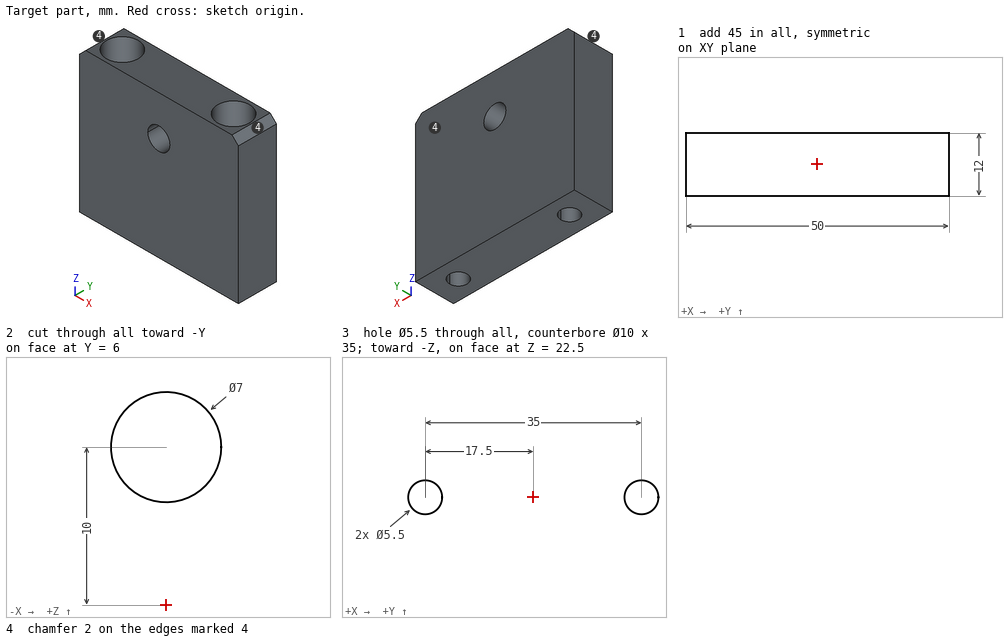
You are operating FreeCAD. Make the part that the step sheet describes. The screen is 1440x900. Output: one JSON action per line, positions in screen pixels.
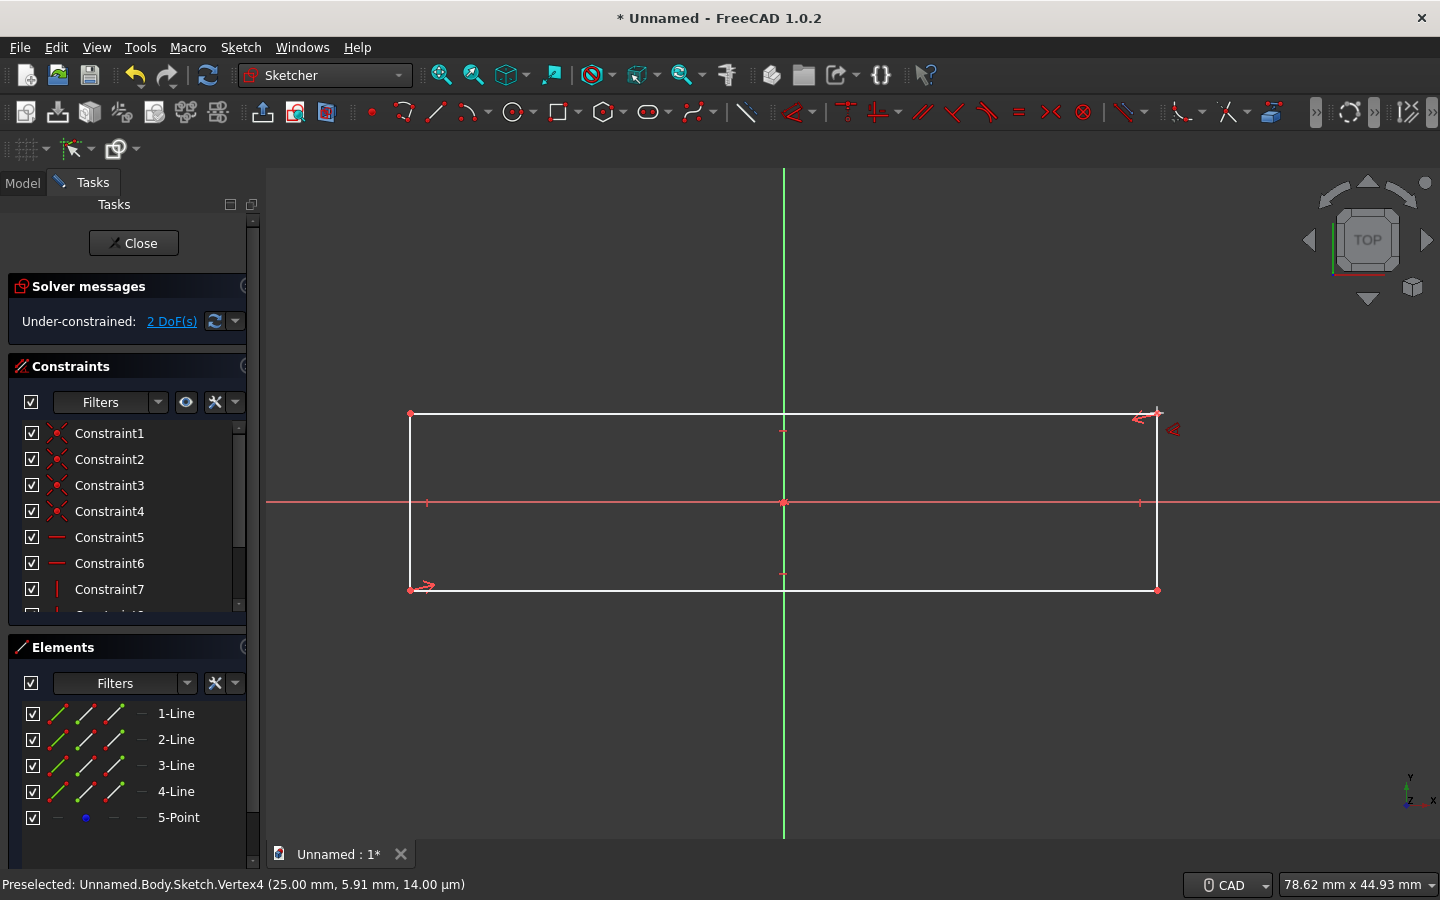
{"action": "left_click", "coordinate": [634, 591]}
{"action": "left_click", "coordinate": [612, 625]}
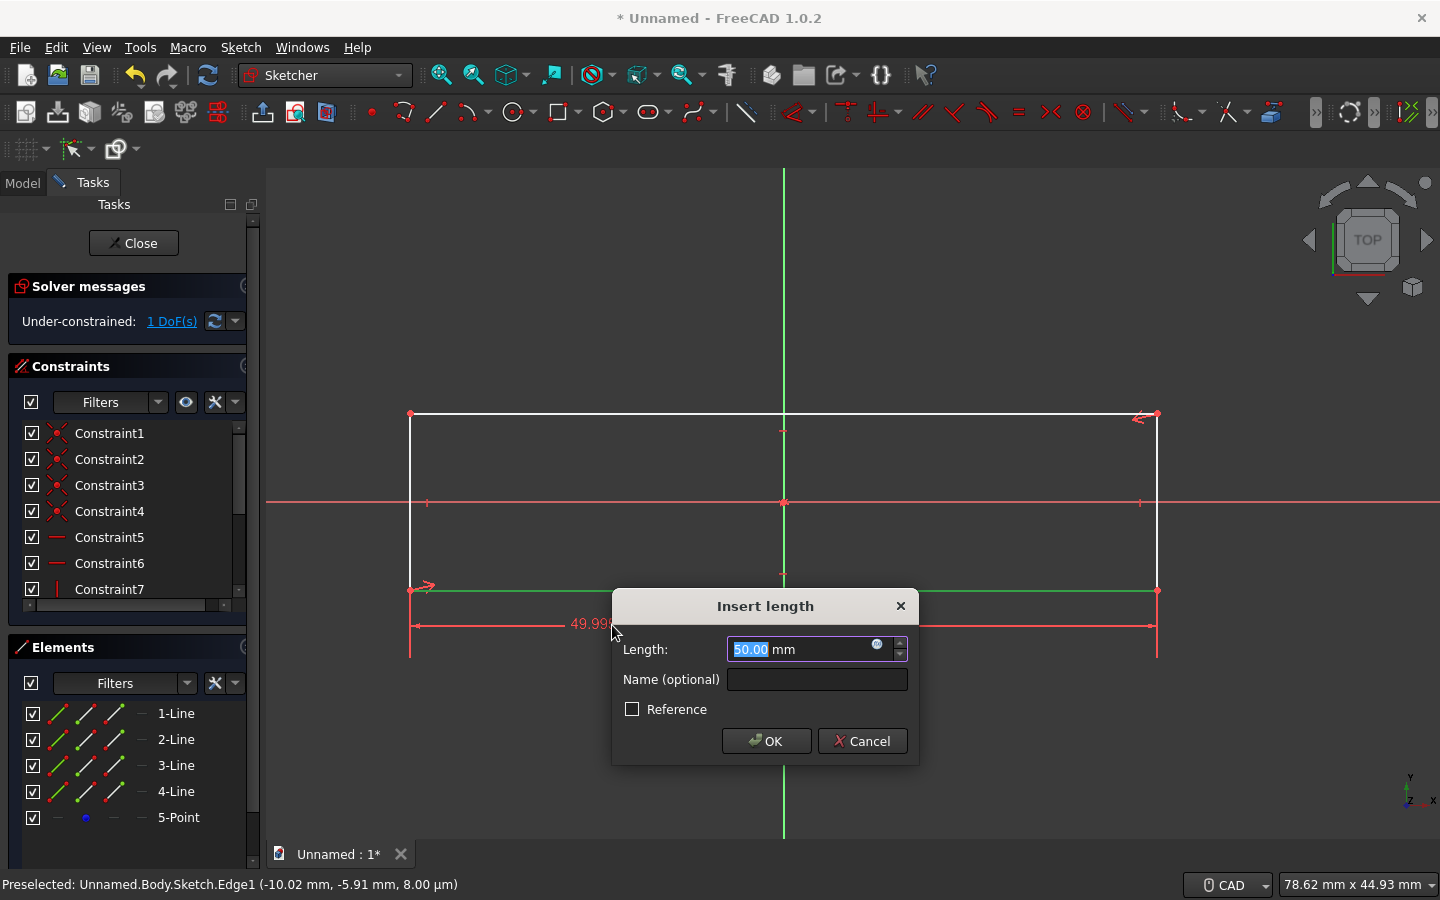
{"action": "type", "text": "50"}
{"action": "key", "text": "Return"}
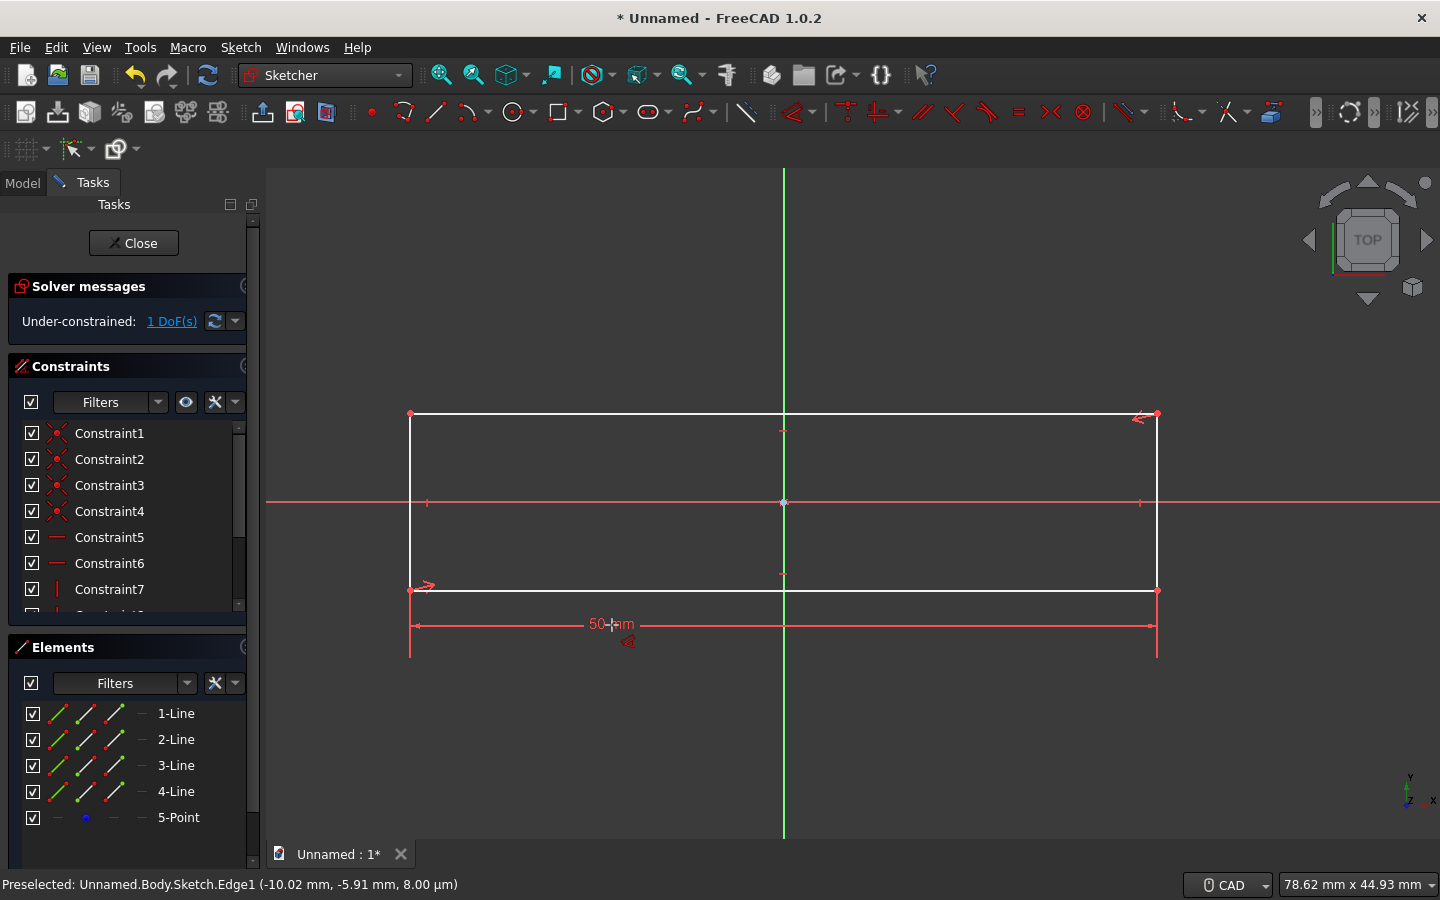
{"action": "left_click", "coordinate": [1157, 538]}
{"action": "left_click", "coordinate": [1191, 462]}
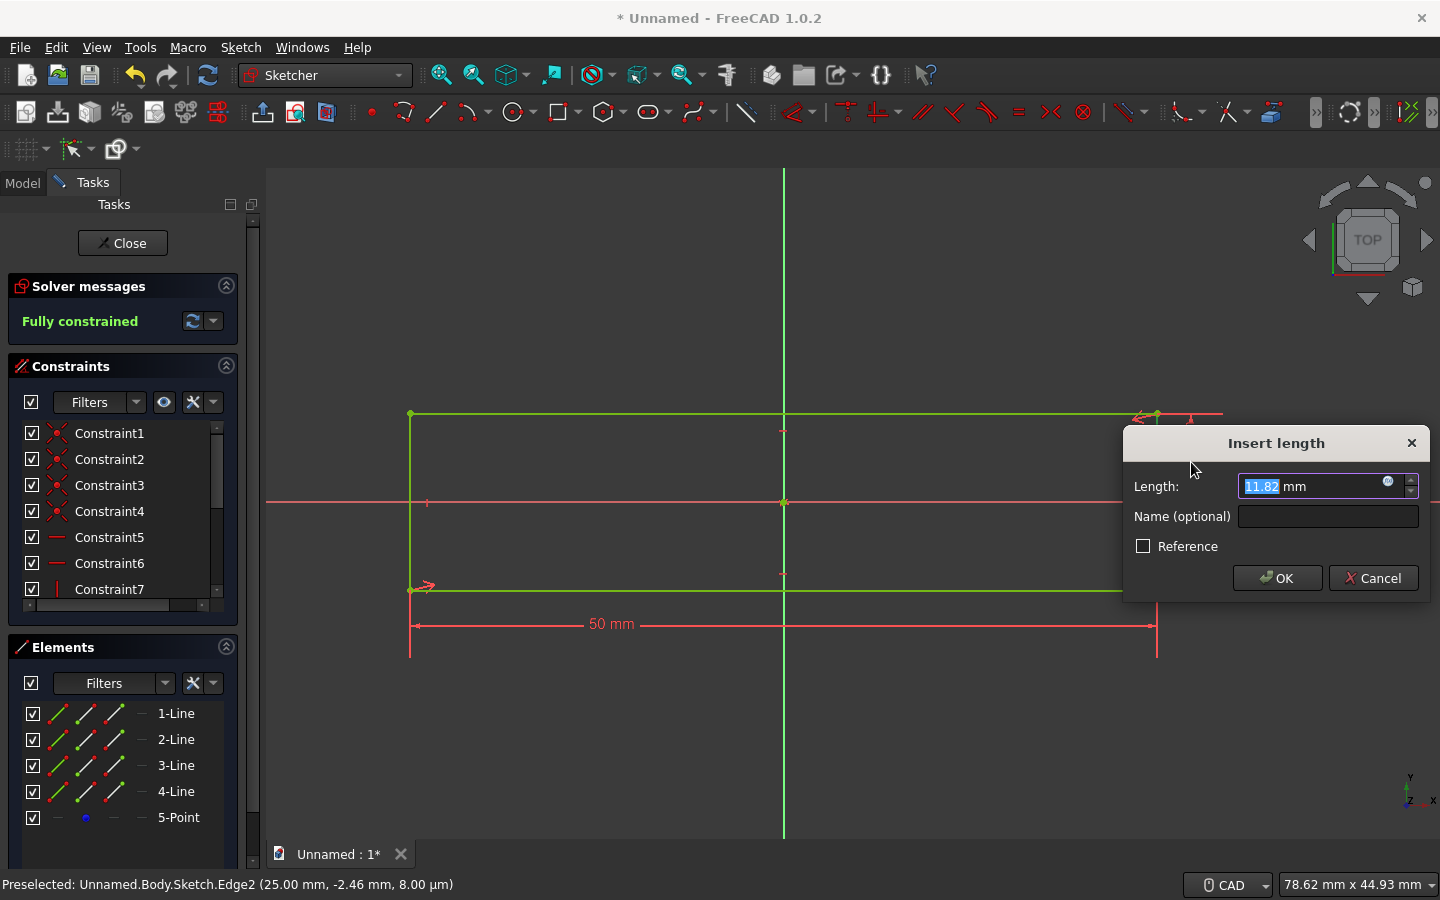
{"action": "type", "text": "12"}
{"action": "key", "text": "Return"}
{"action": "key", "text": "Escape"}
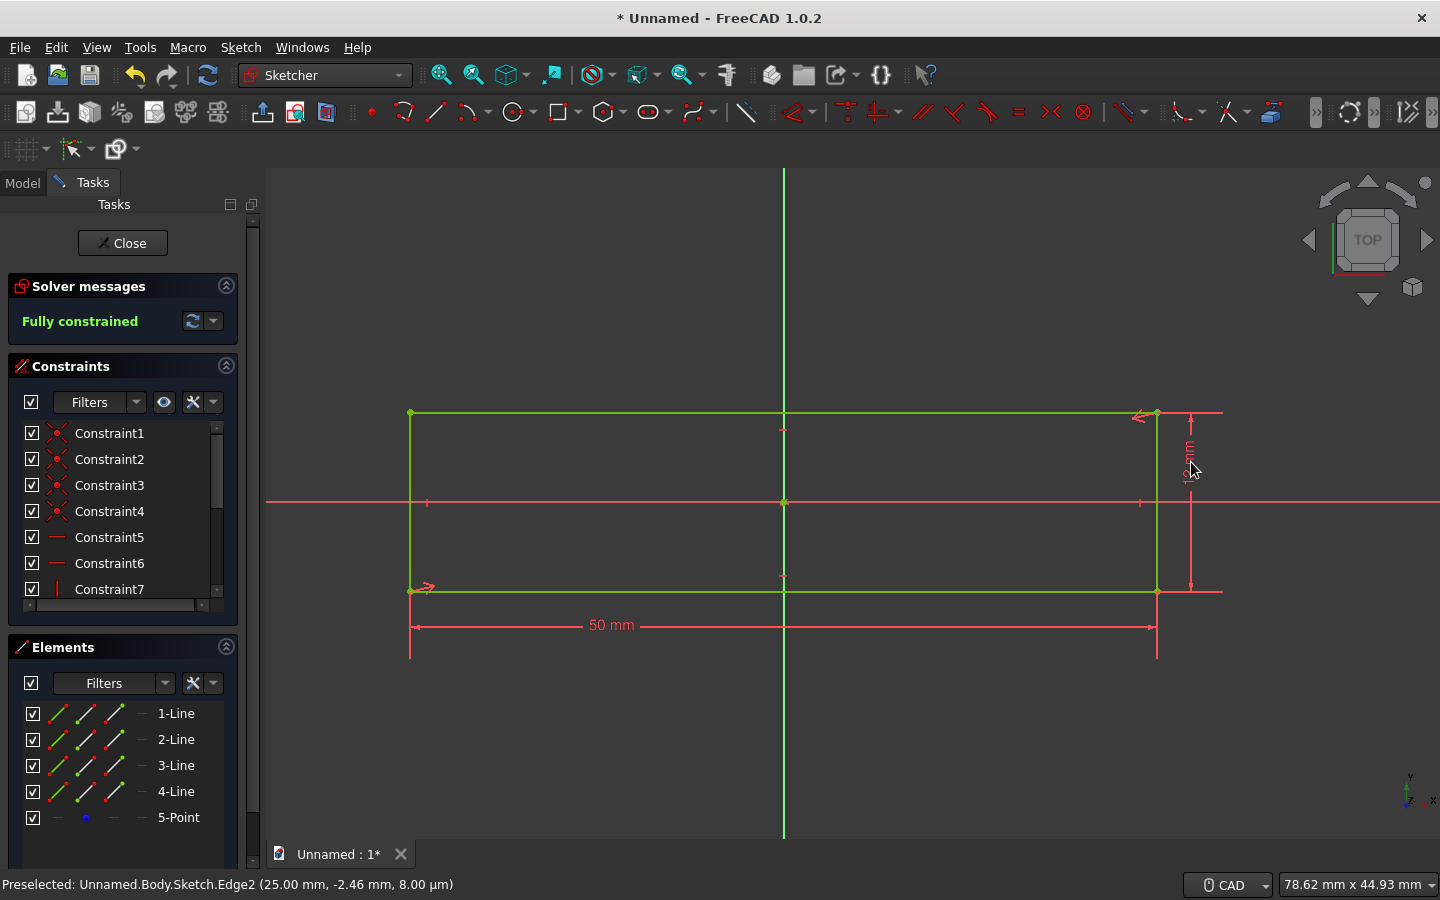
{"action": "left_click", "coordinate": [123, 243]}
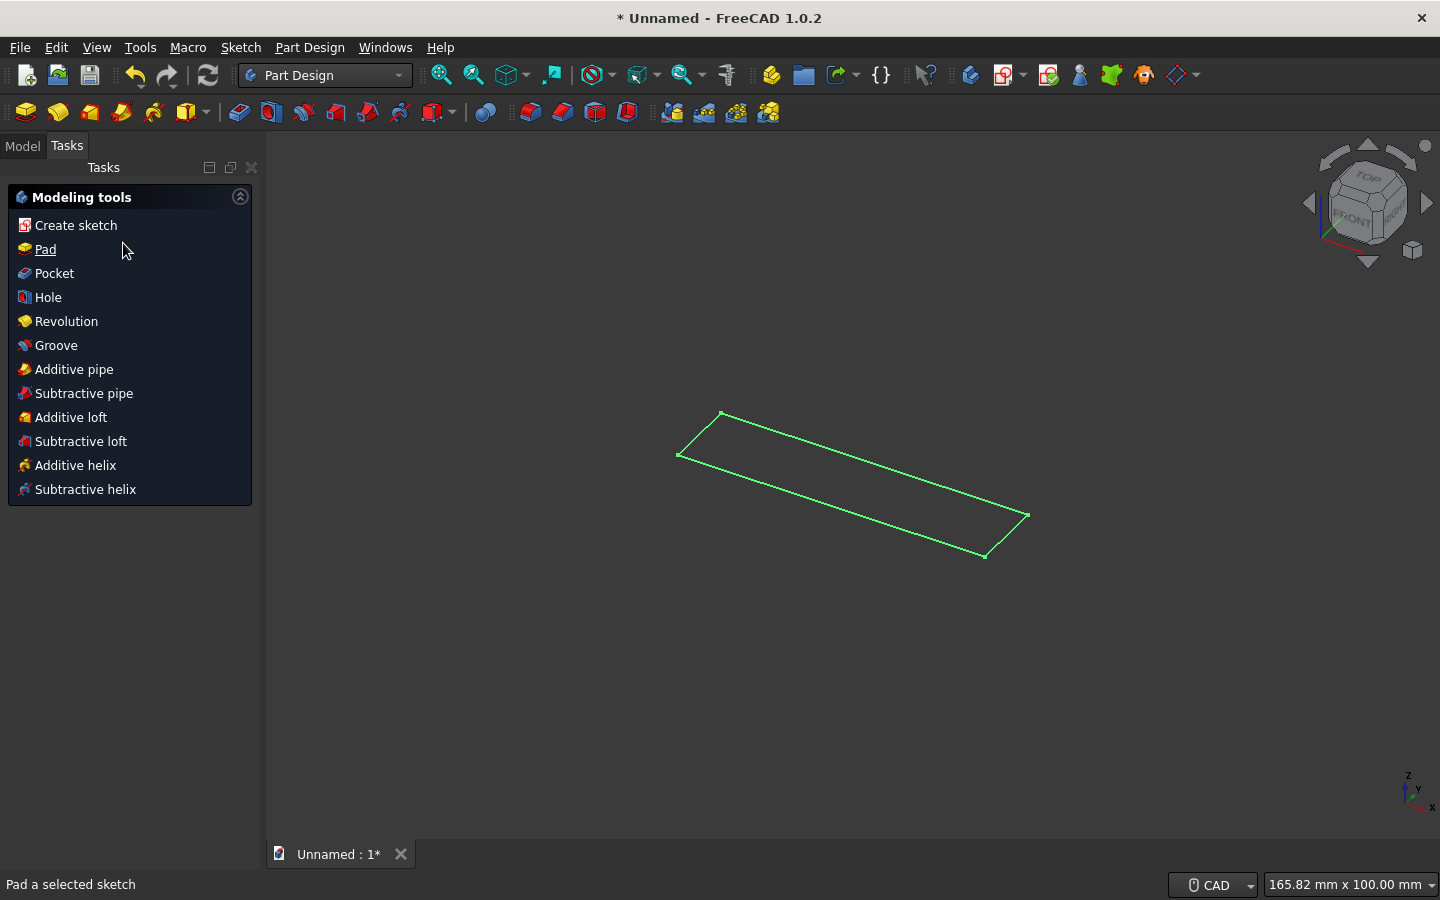
{"action": "left_click", "coordinate": [26, 112]}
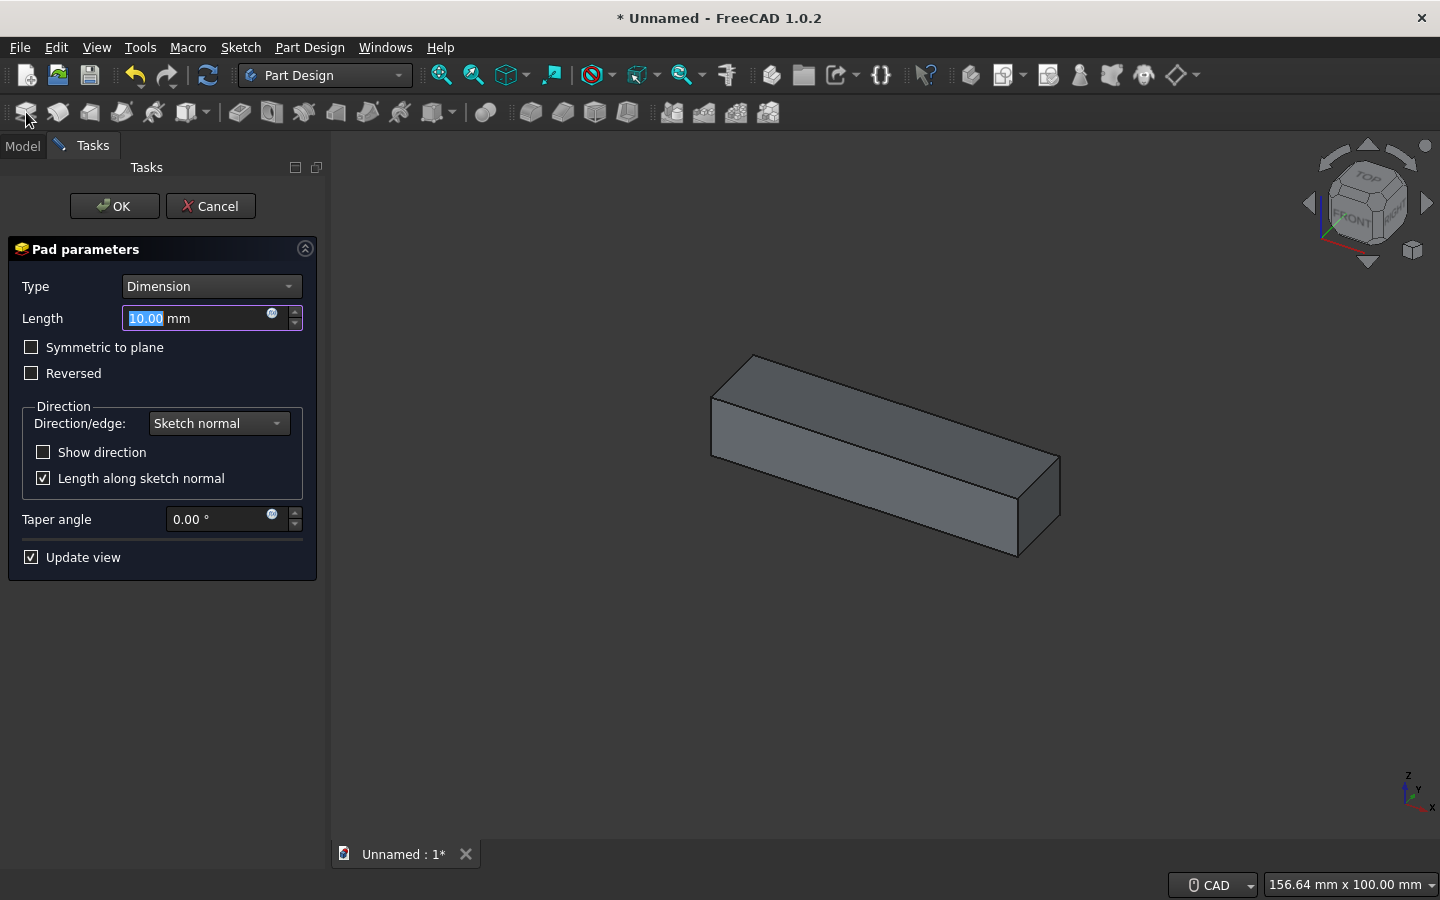
{"action": "type", "text": "45"}
{"action": "key", "text": "Tab"}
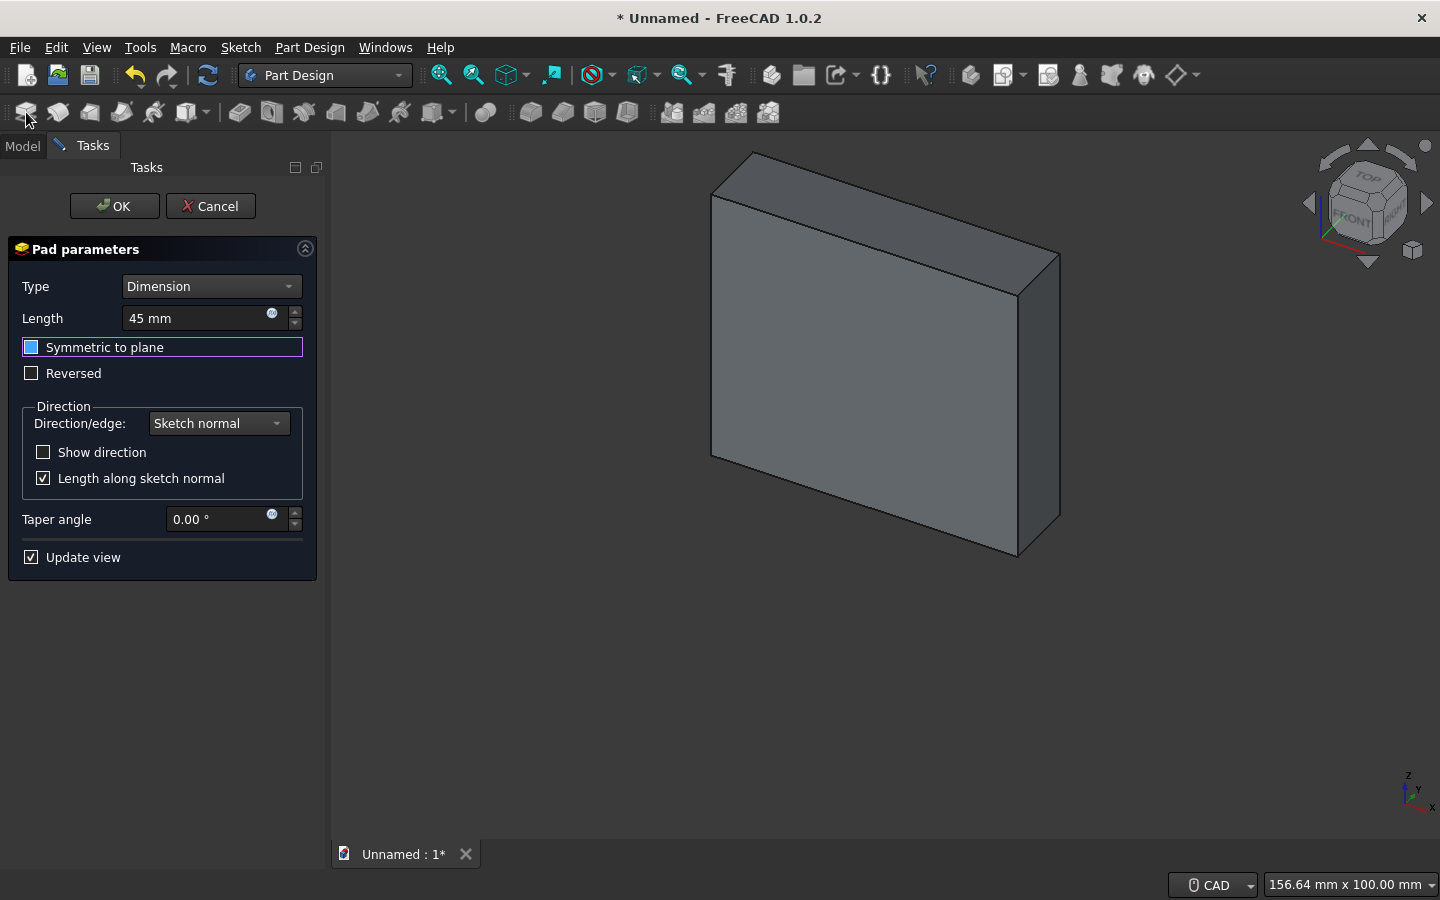
{"action": "left_click", "coordinate": [30, 347]}